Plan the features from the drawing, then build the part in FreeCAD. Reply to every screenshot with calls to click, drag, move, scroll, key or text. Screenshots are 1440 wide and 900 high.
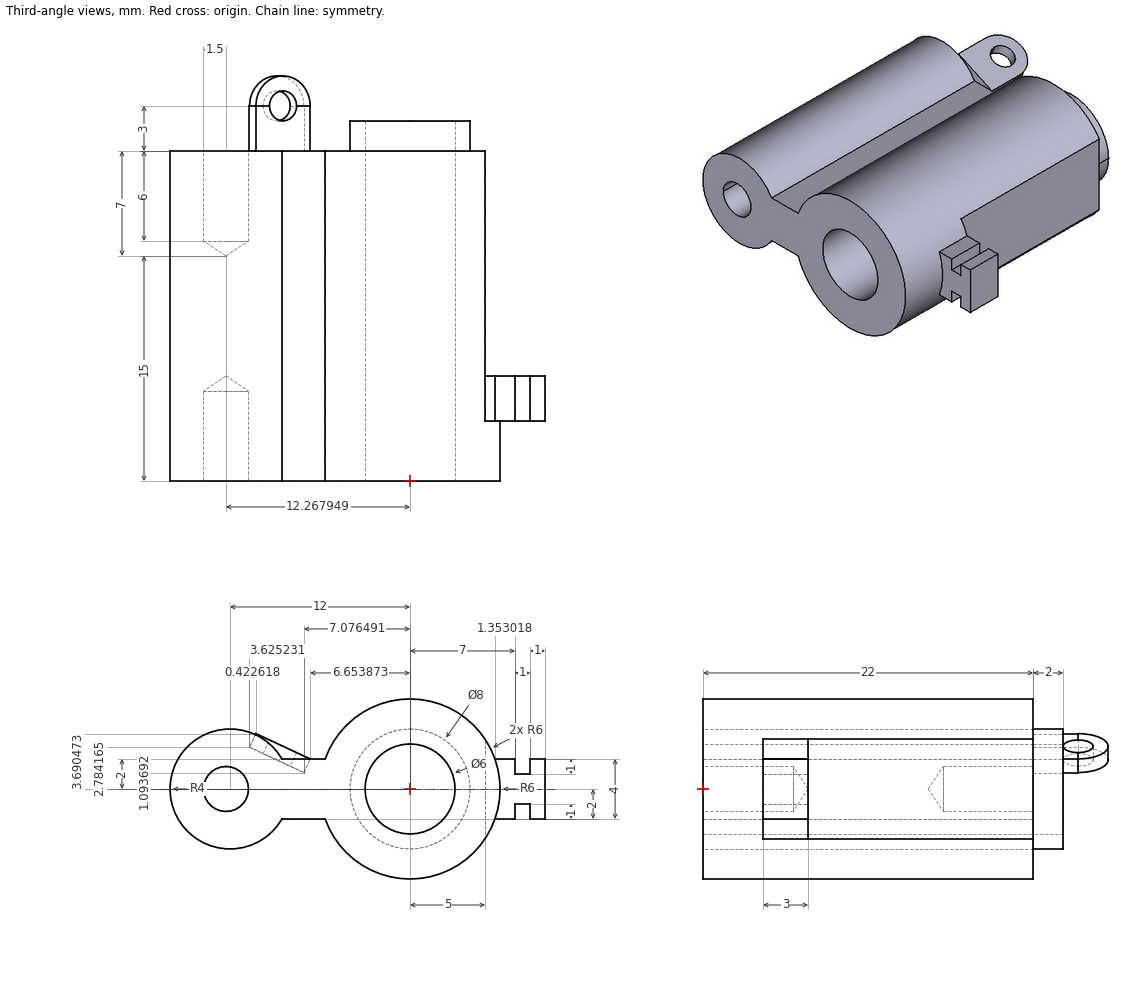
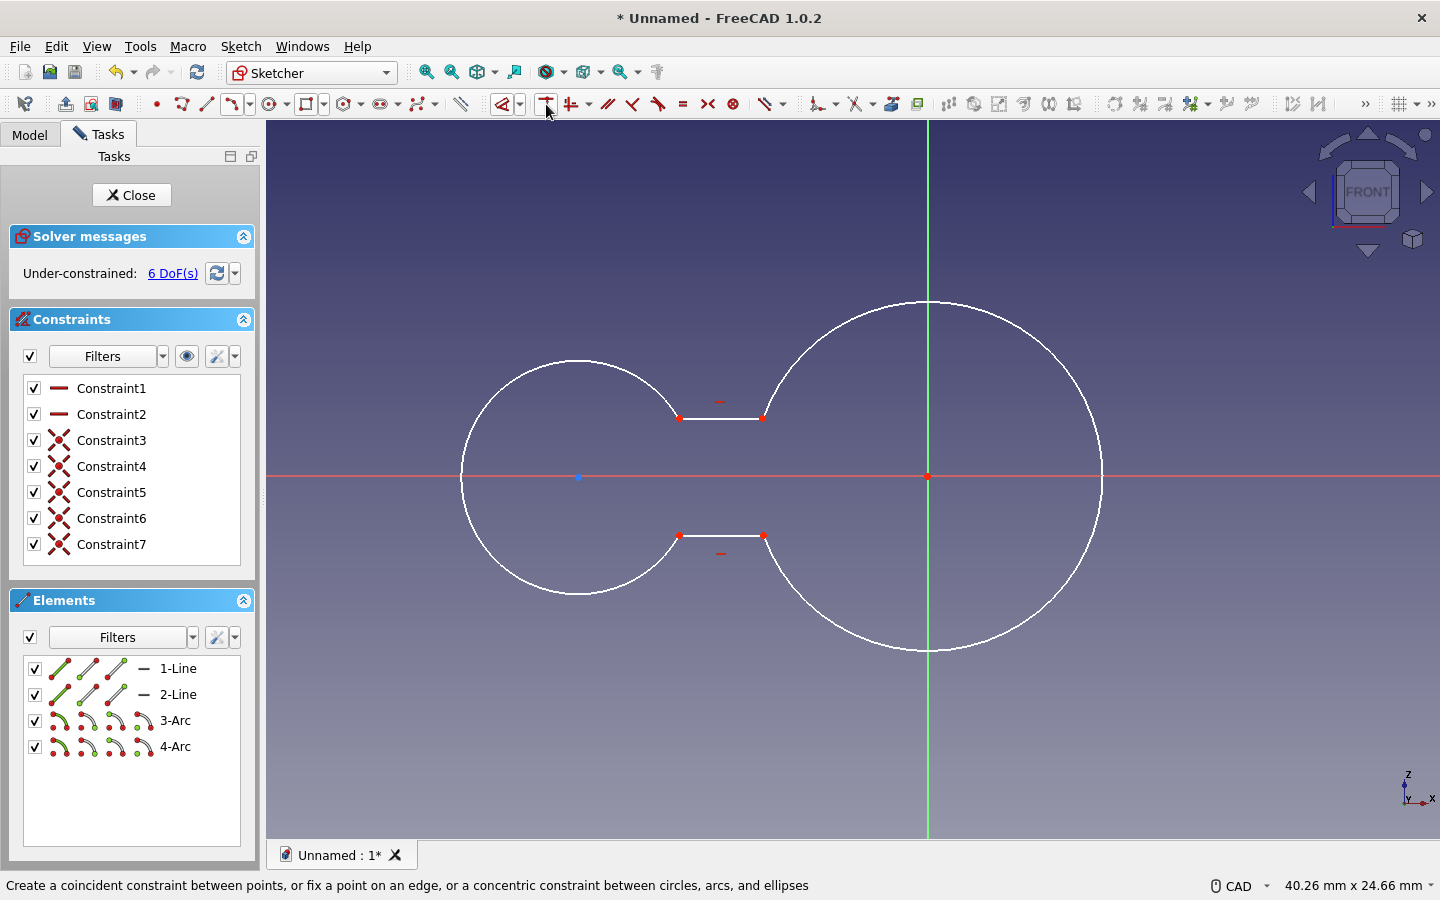
click(578, 477)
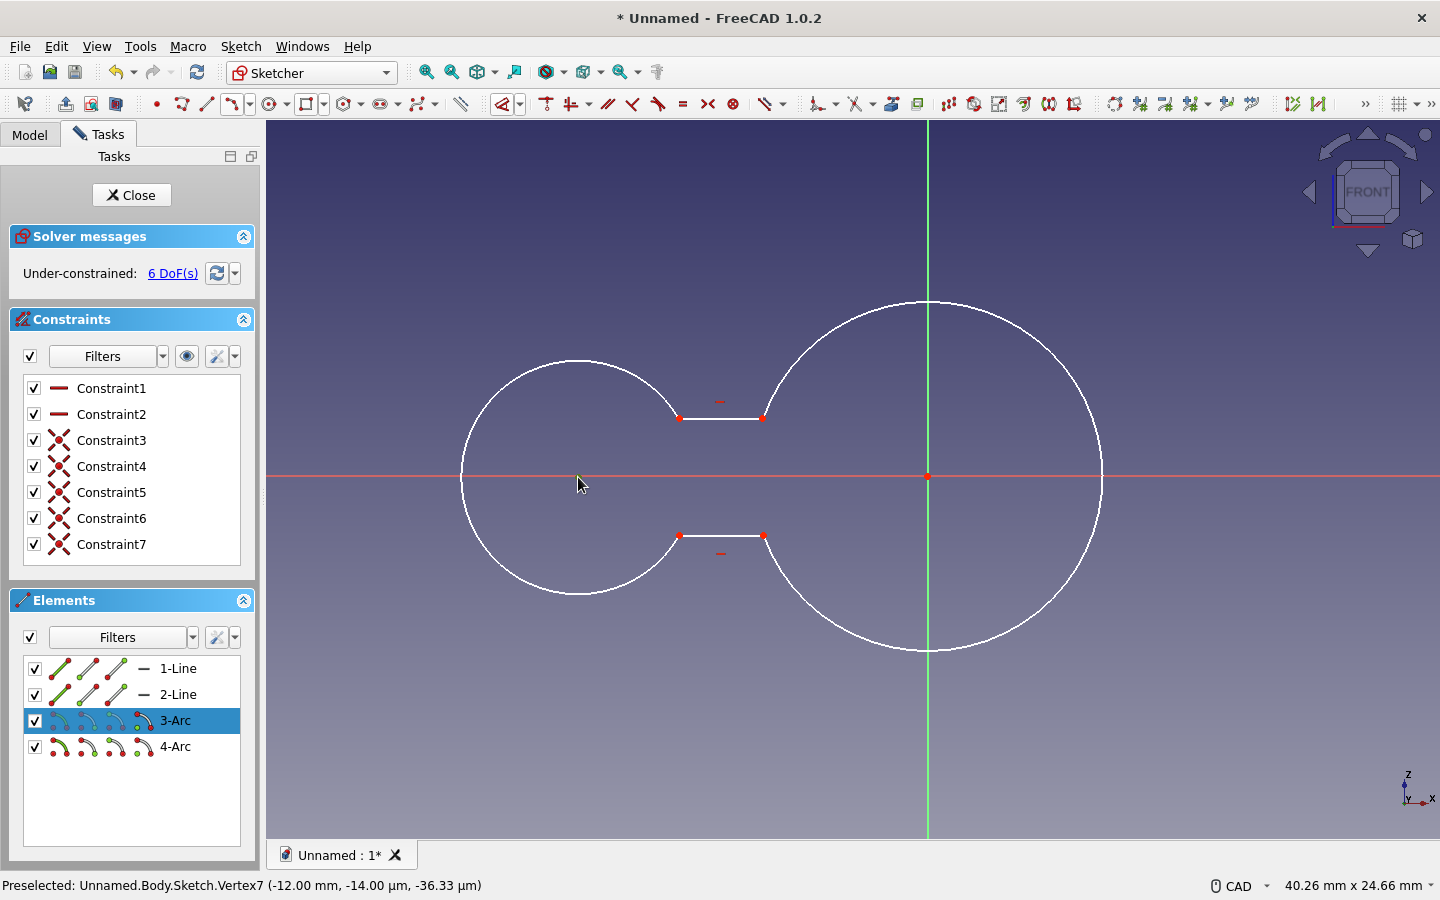
click(364, 476)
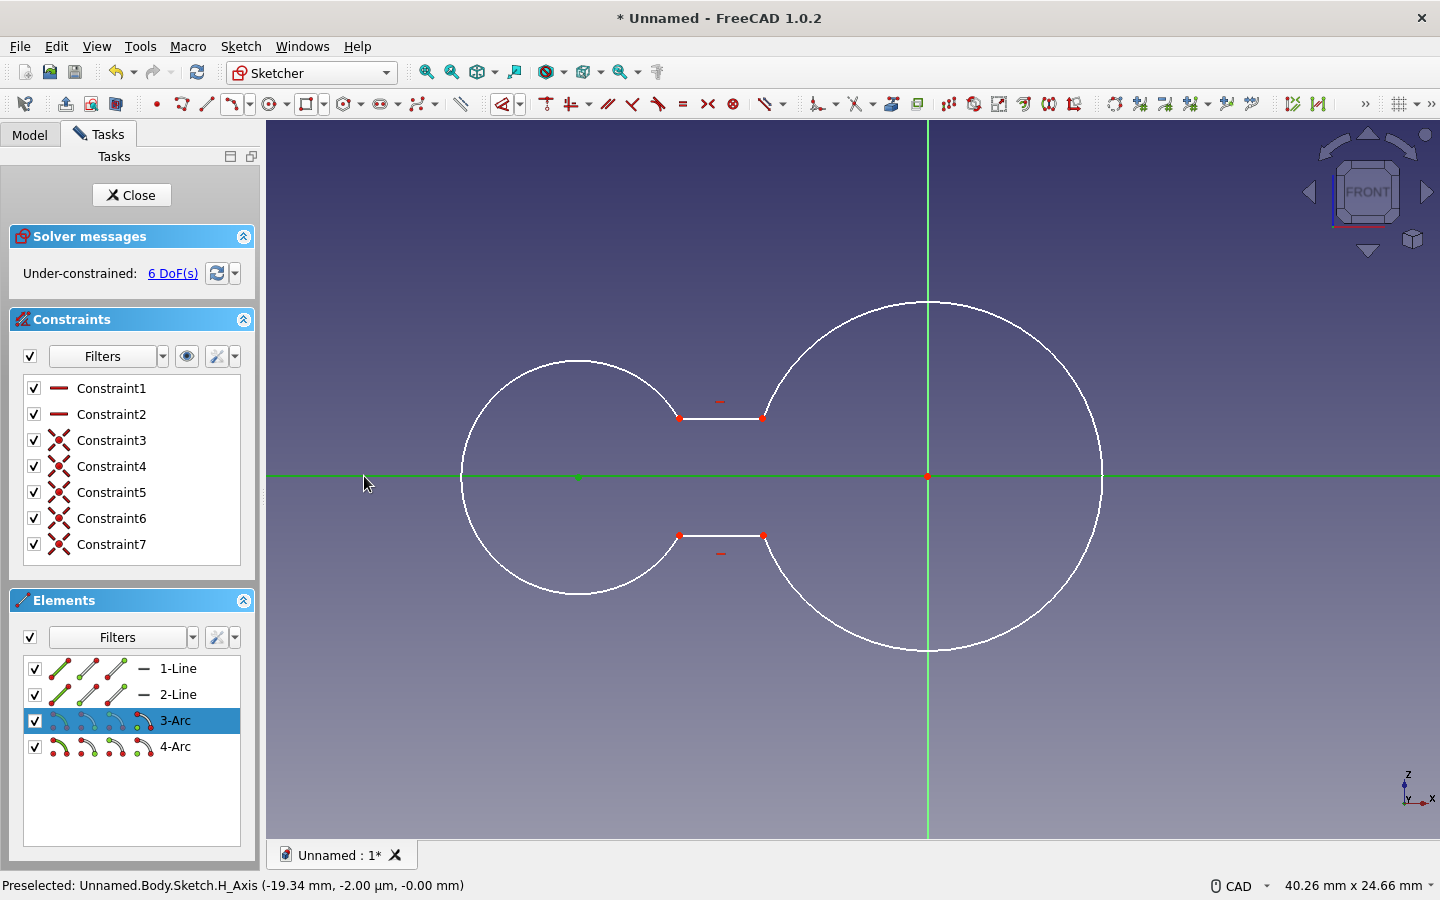
click(546, 104)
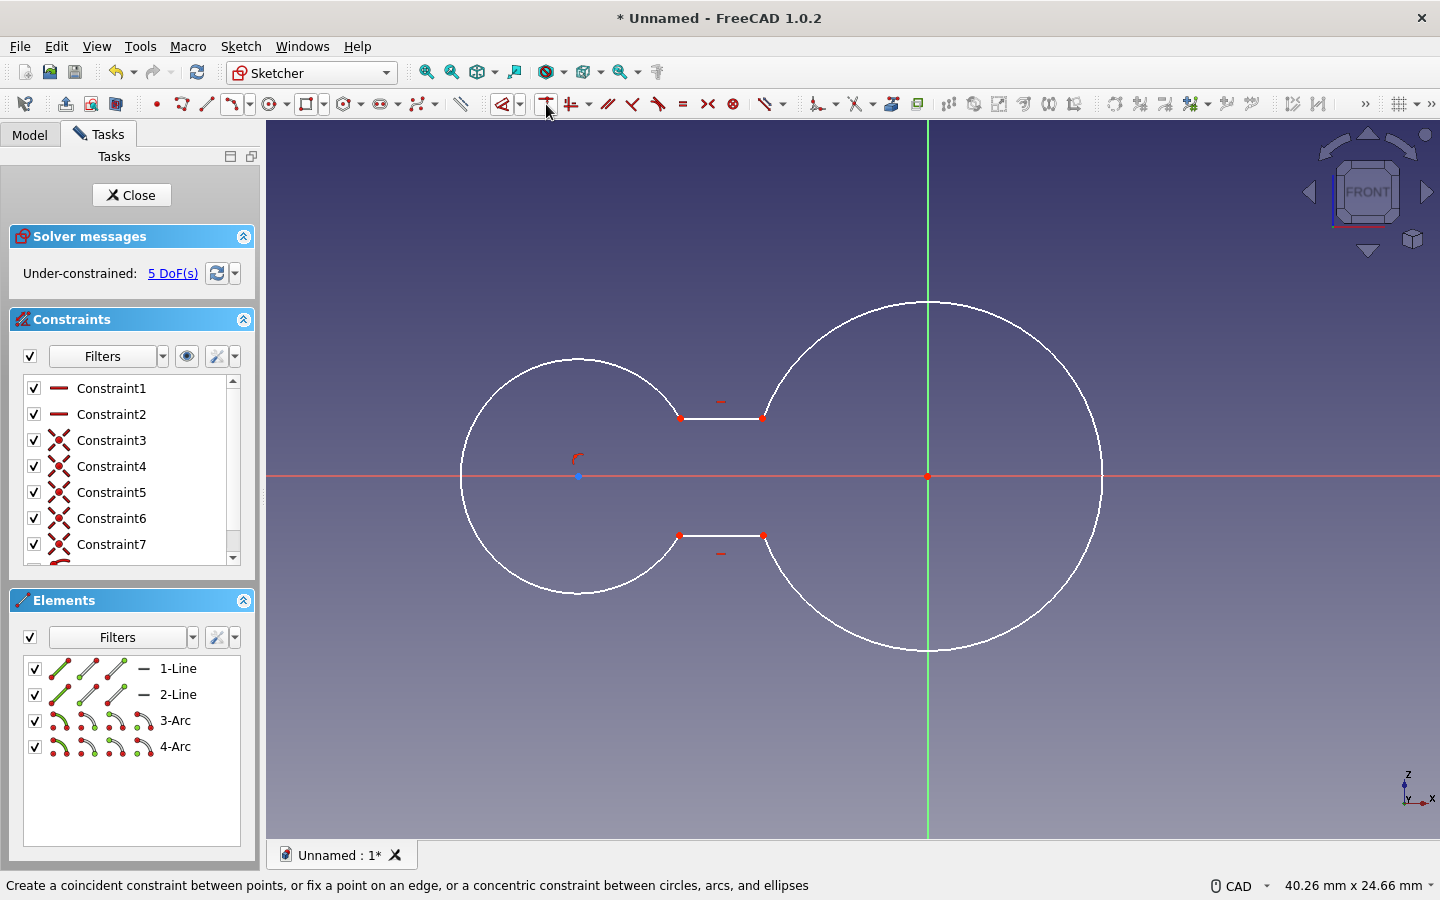
click(502, 104)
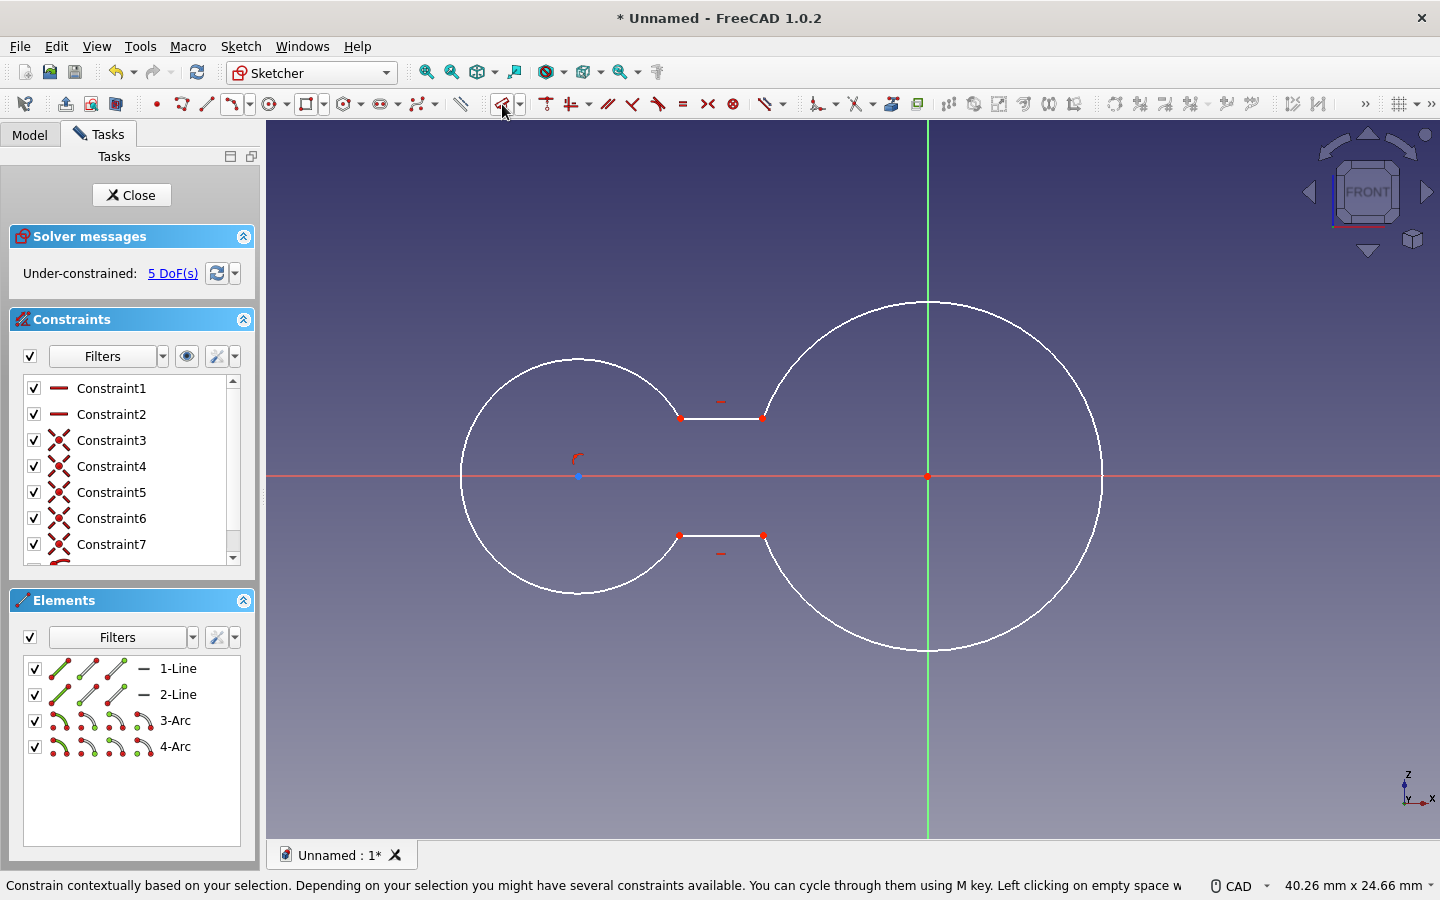
click(520, 374)
click(504, 346)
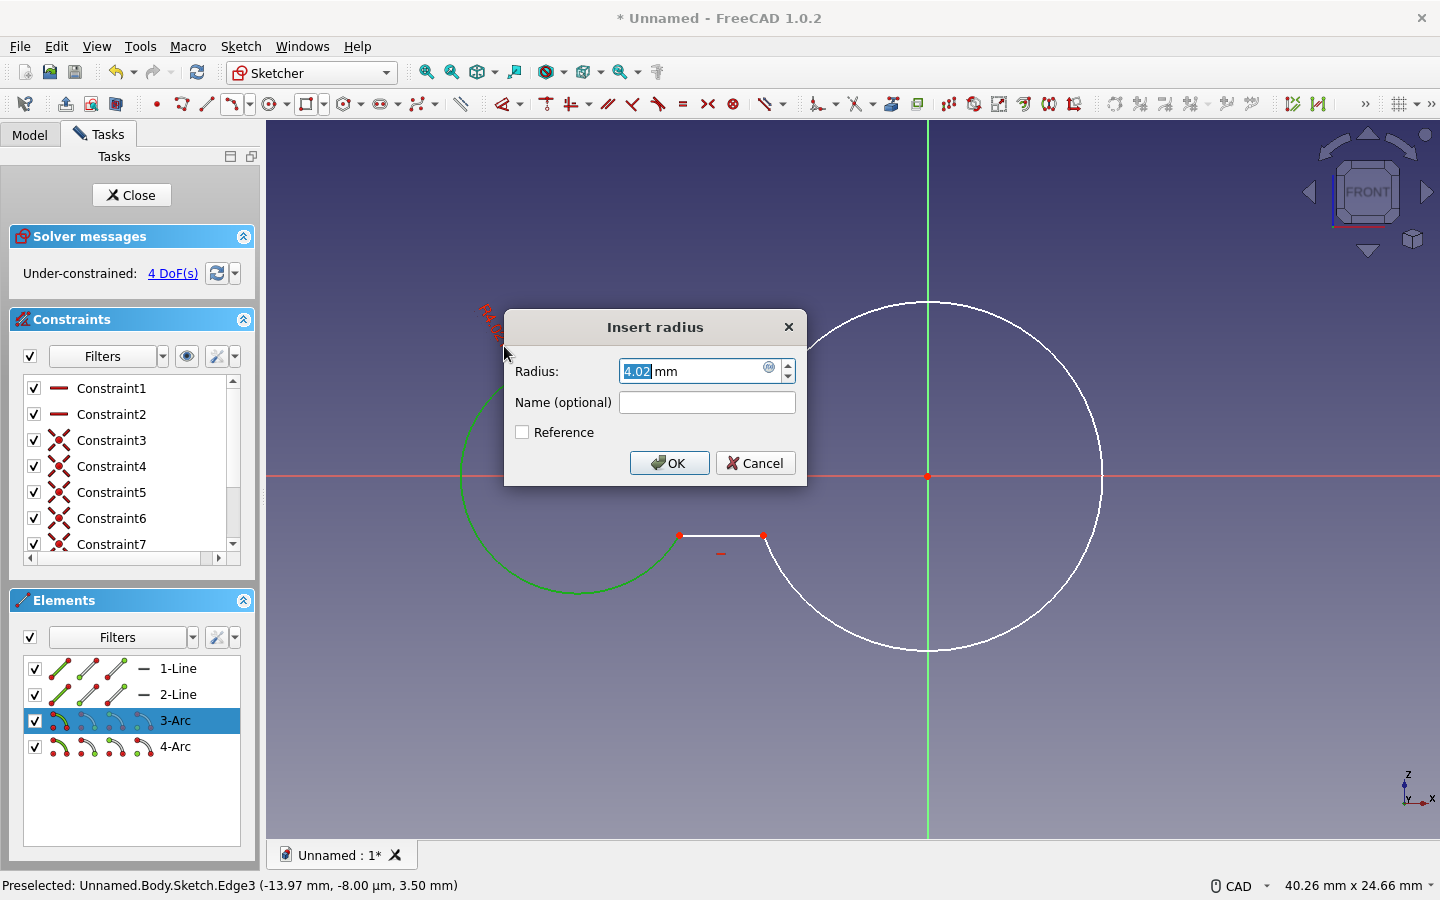
text(4)
key(Return)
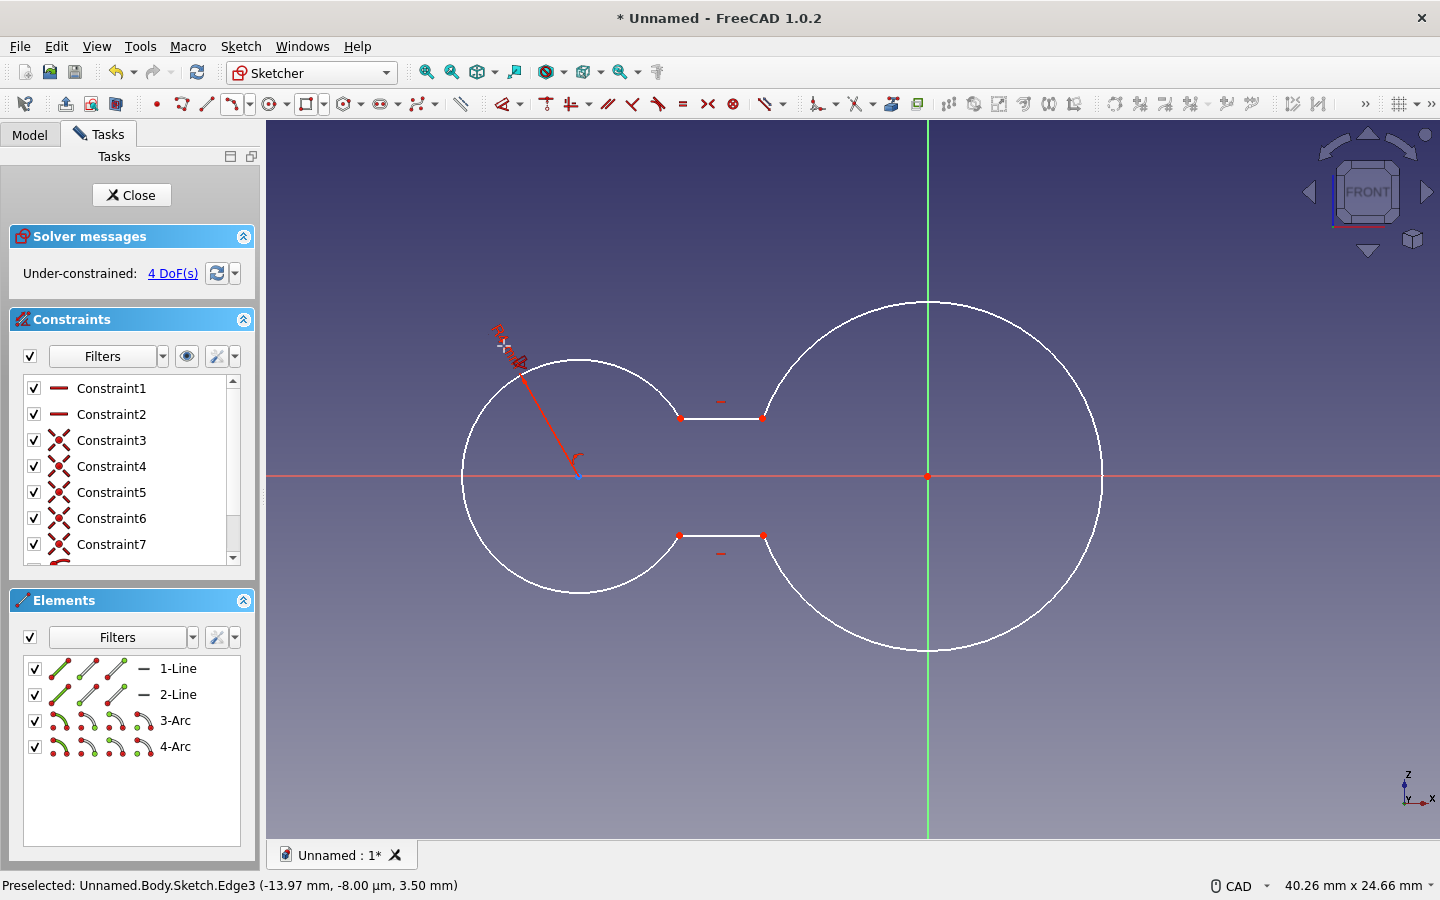
click(1005, 633)
click(1019, 662)